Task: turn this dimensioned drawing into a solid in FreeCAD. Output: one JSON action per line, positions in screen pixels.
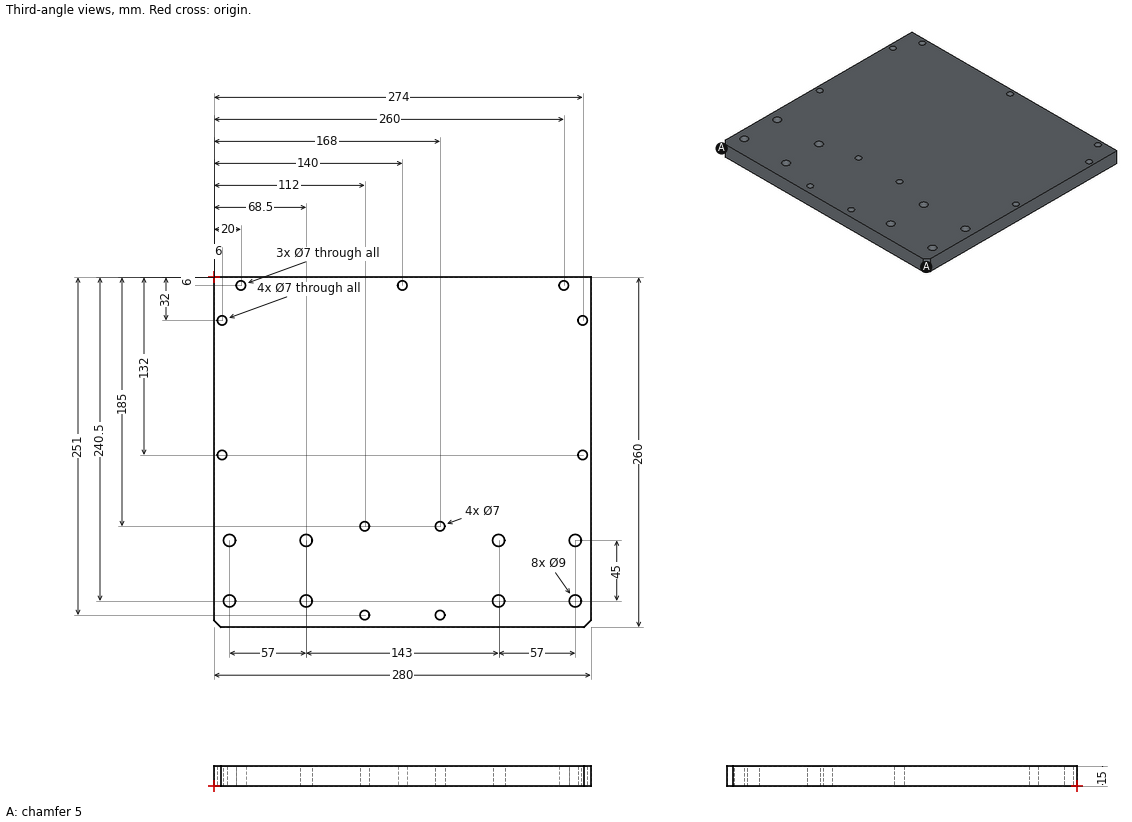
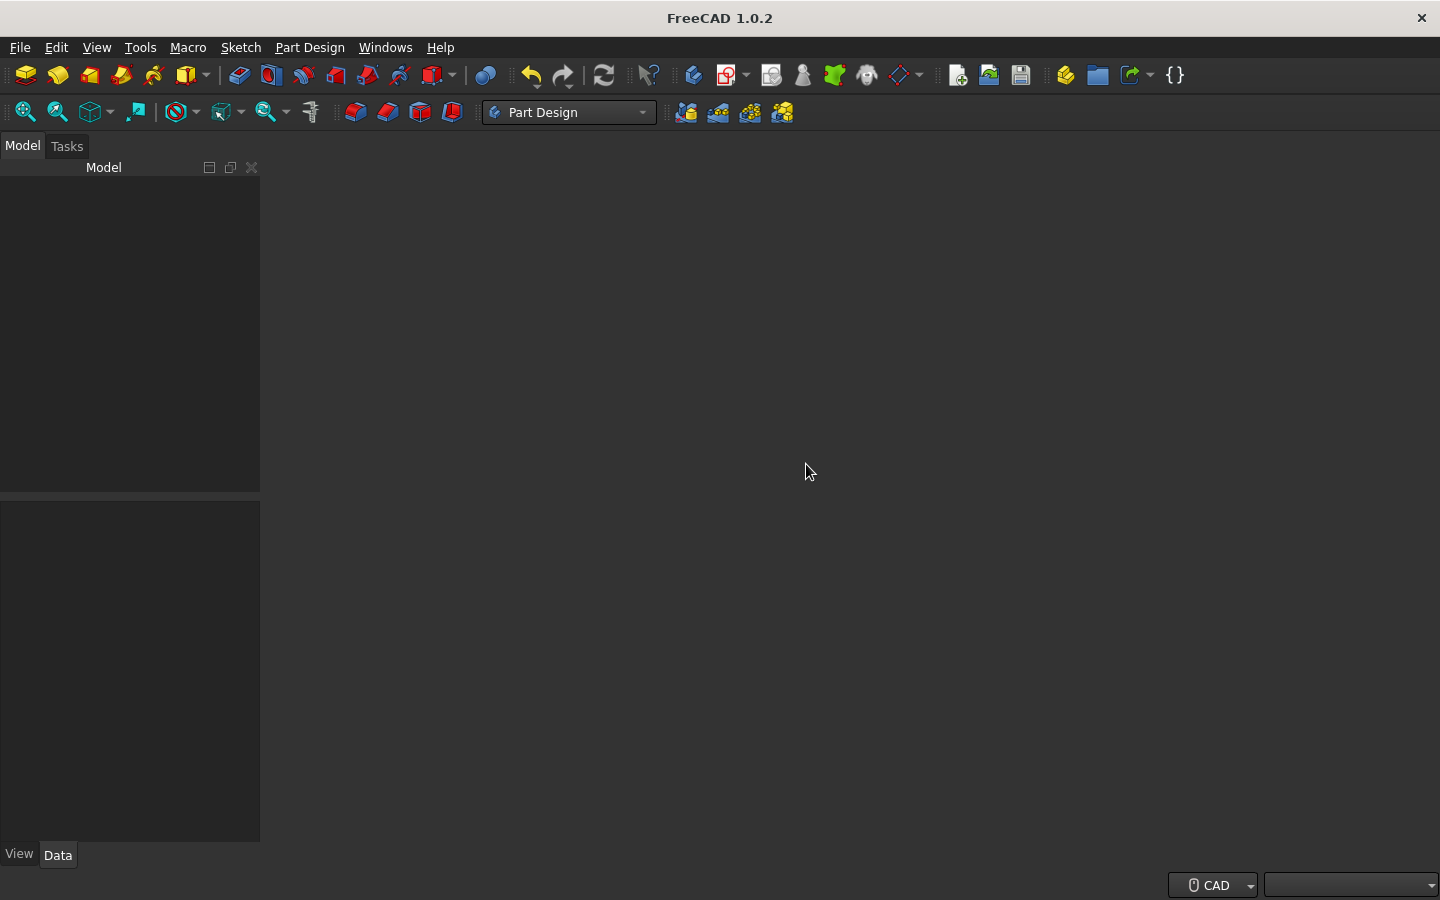
{"action": "left_click", "coordinate": [958, 76]}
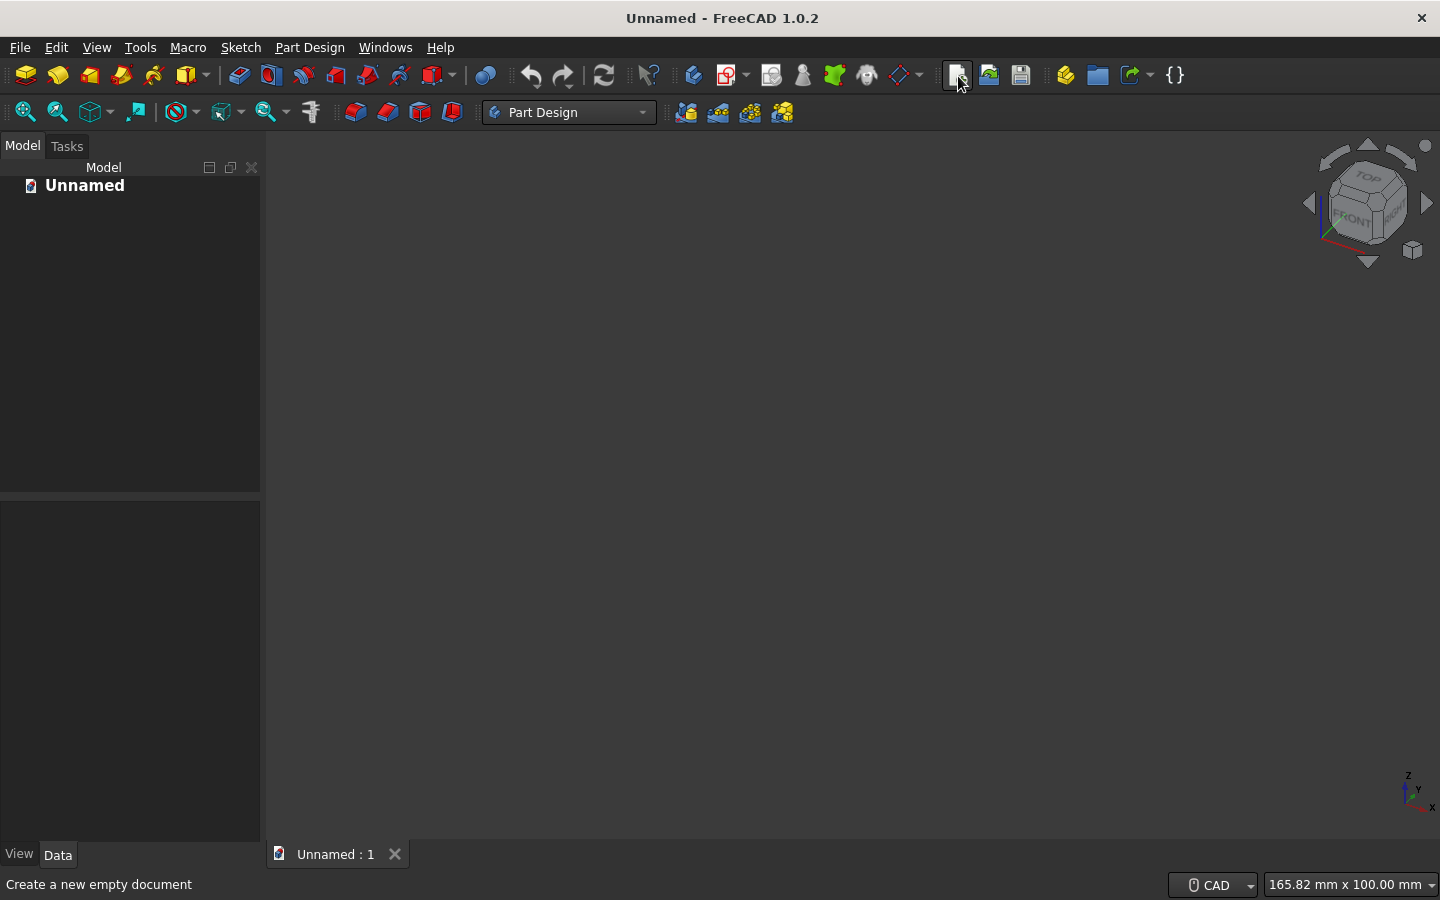
{"action": "left_click", "coordinate": [726, 76]}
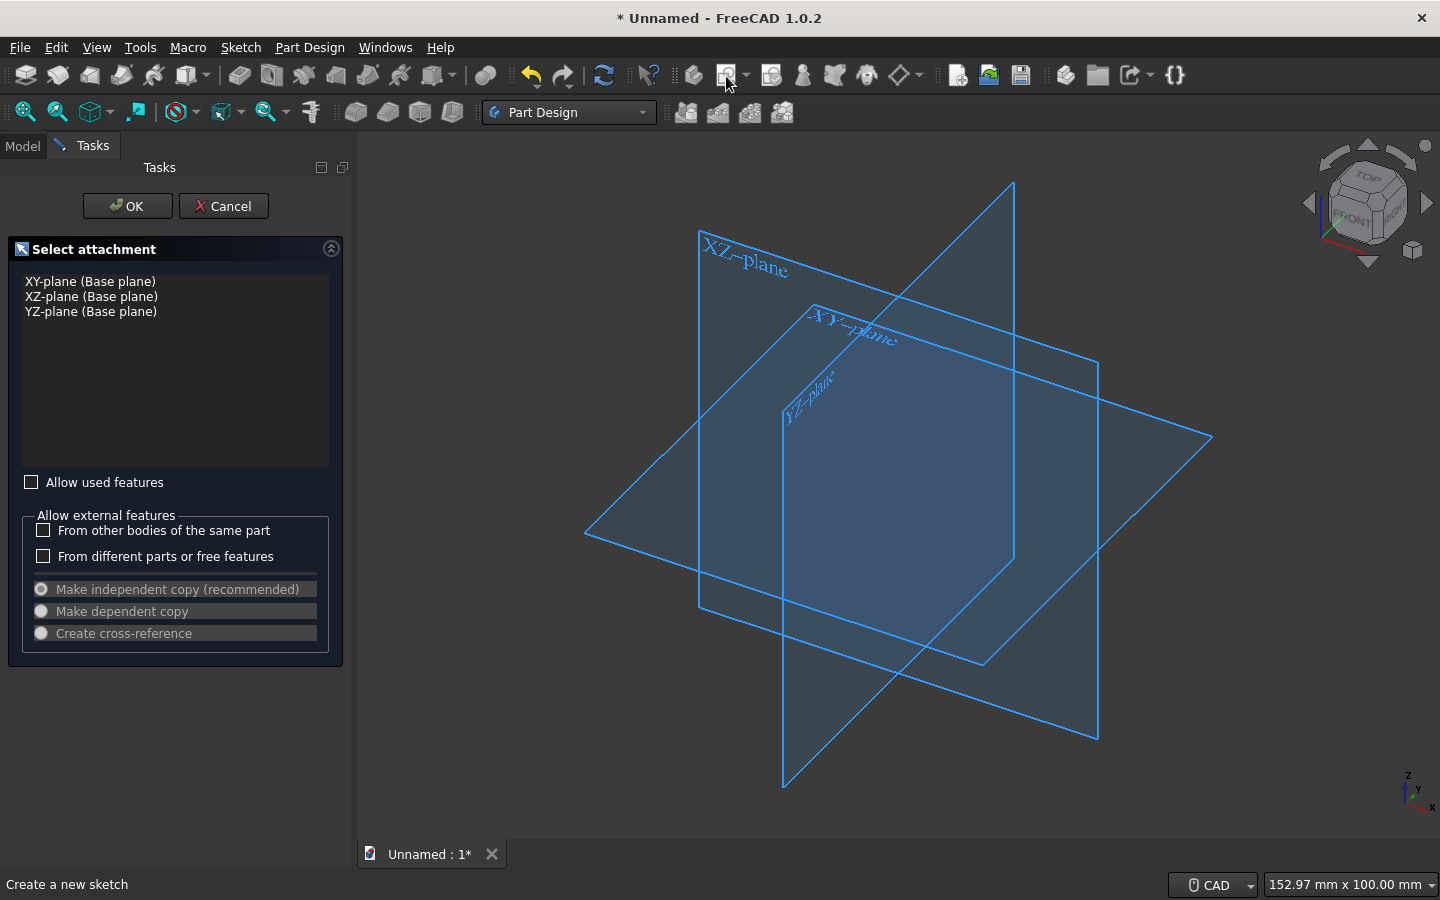
{"action": "left_click", "coordinate": [82, 282]}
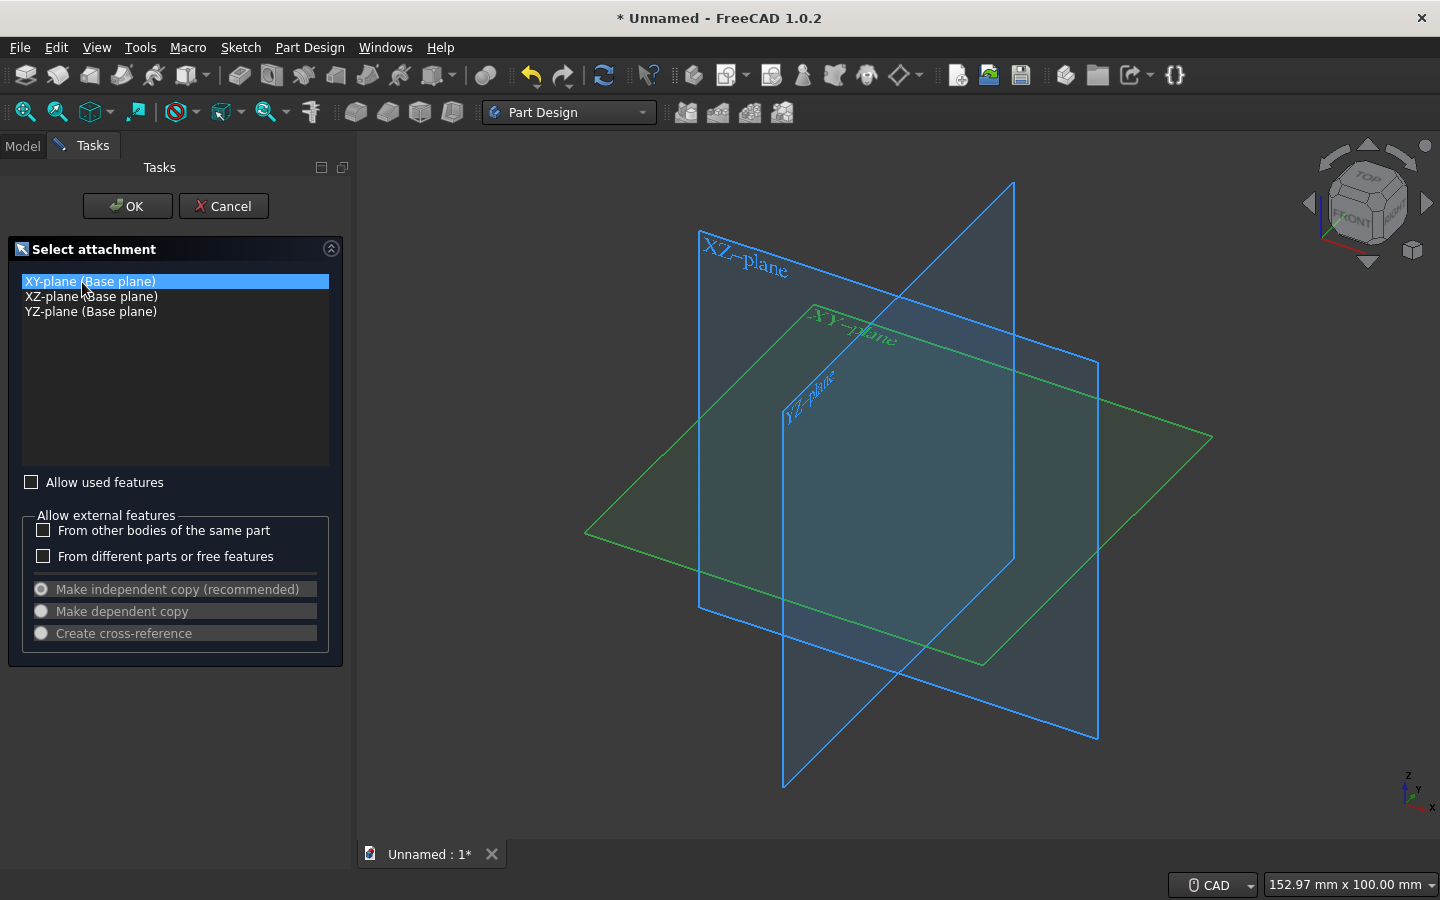
{"action": "left_click", "coordinate": [128, 206]}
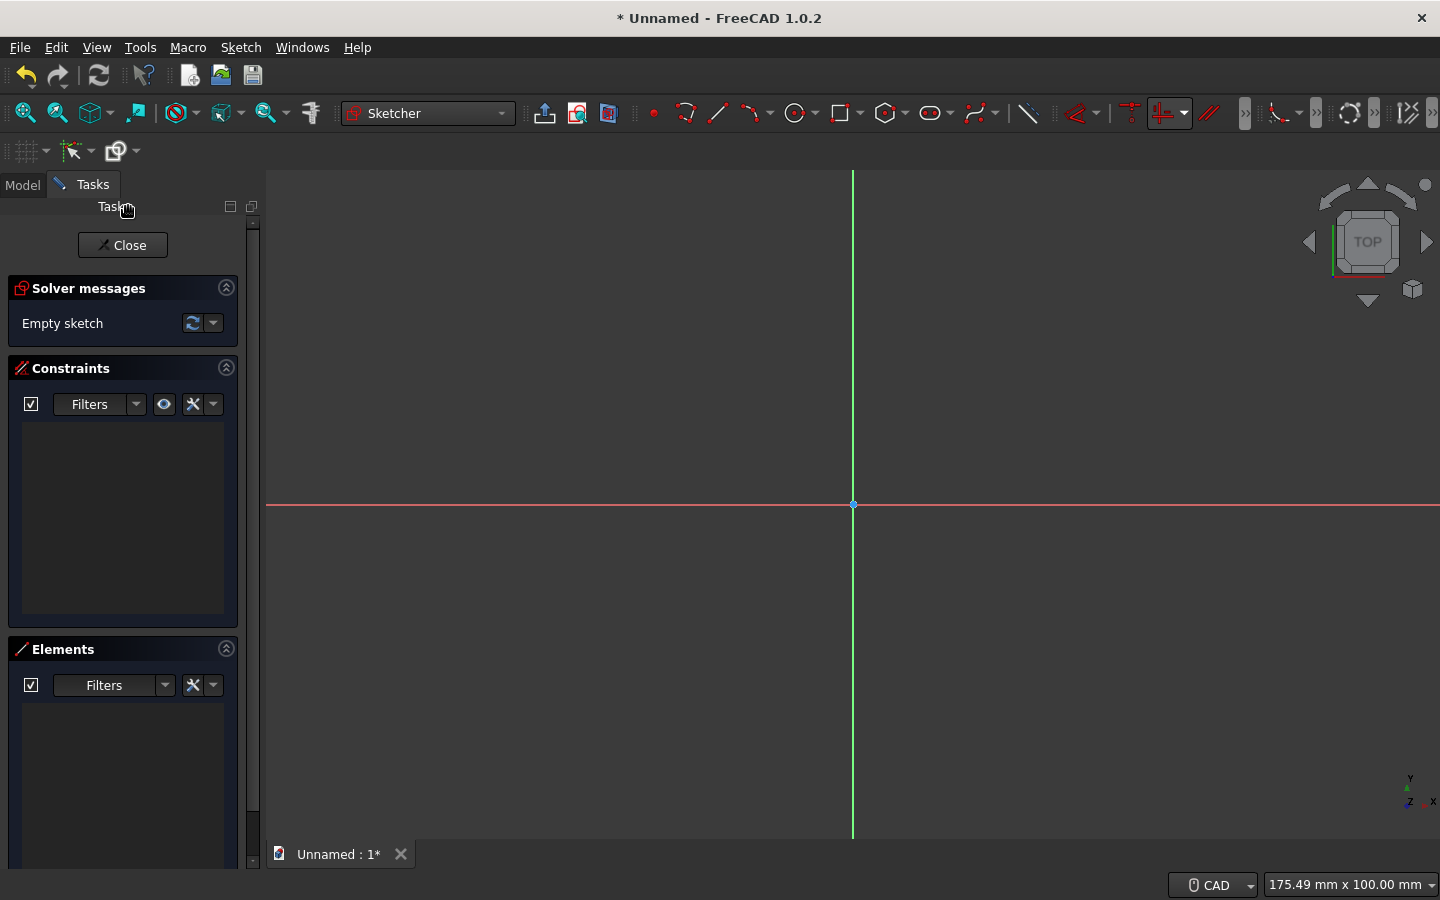
{"action": "scroll", "coordinate": [456, 220], "scroll_direction": "down", "scroll_amount": 7}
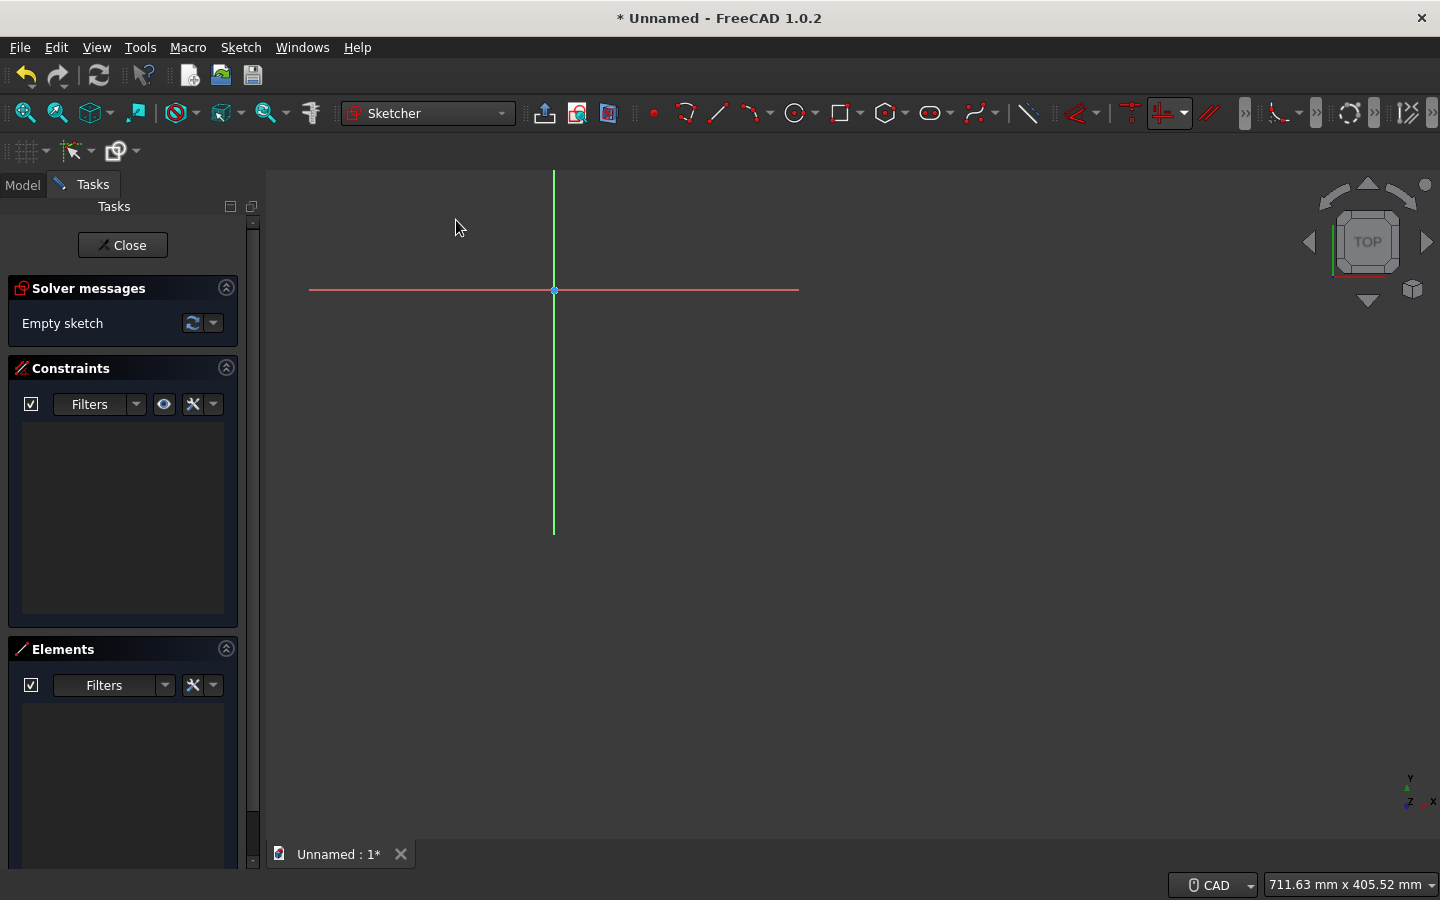
{"action": "left_click", "coordinate": [840, 114]}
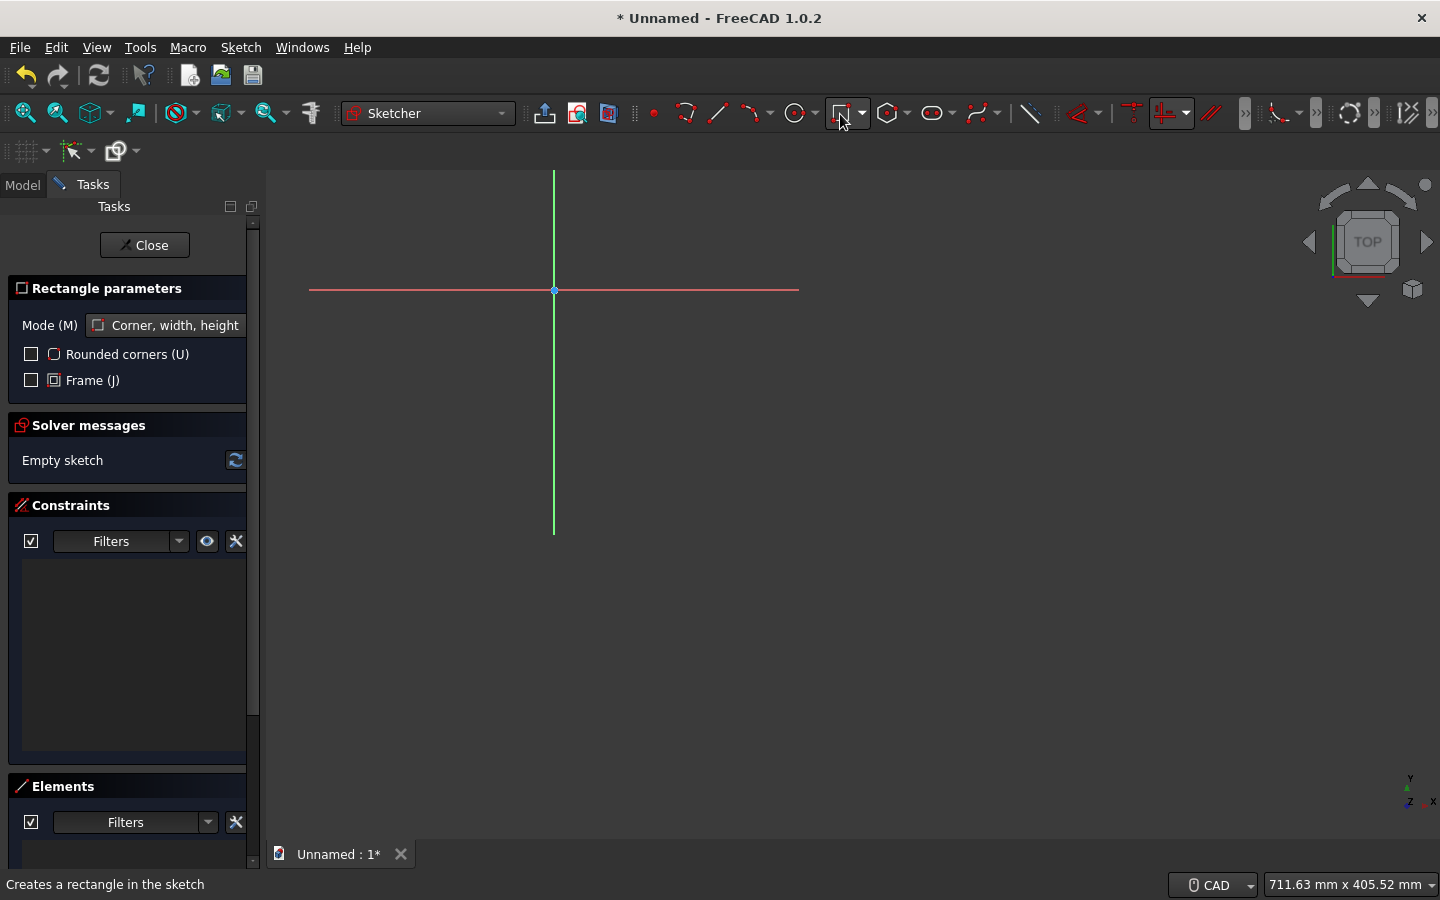
{"action": "left_click", "coordinate": [554, 290]}
{"action": "mouse_move", "coordinate": [1016, 719]}